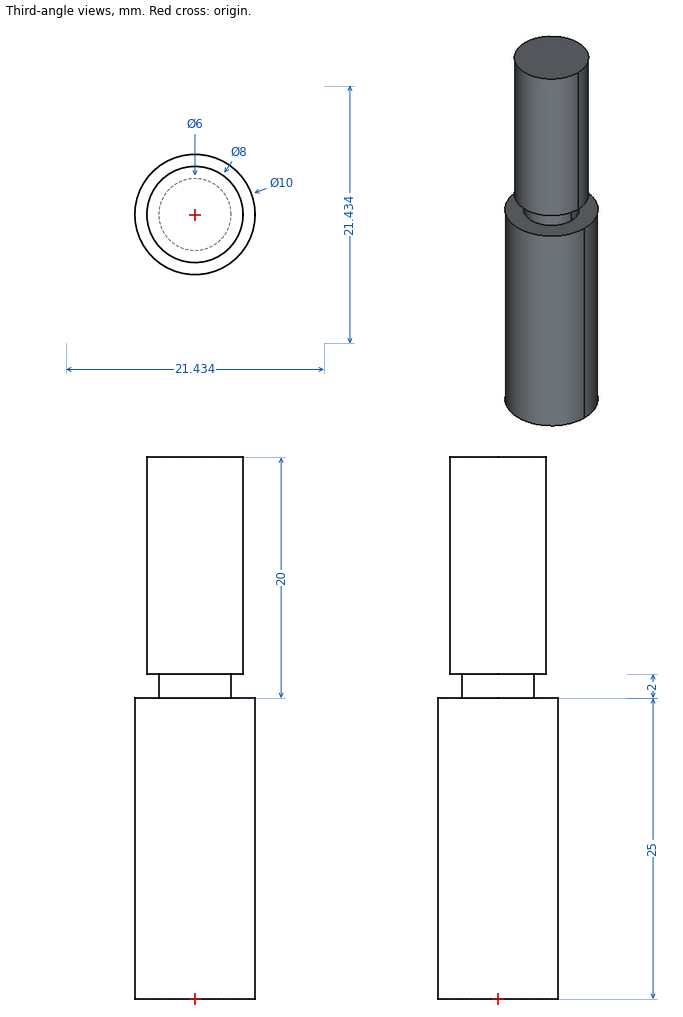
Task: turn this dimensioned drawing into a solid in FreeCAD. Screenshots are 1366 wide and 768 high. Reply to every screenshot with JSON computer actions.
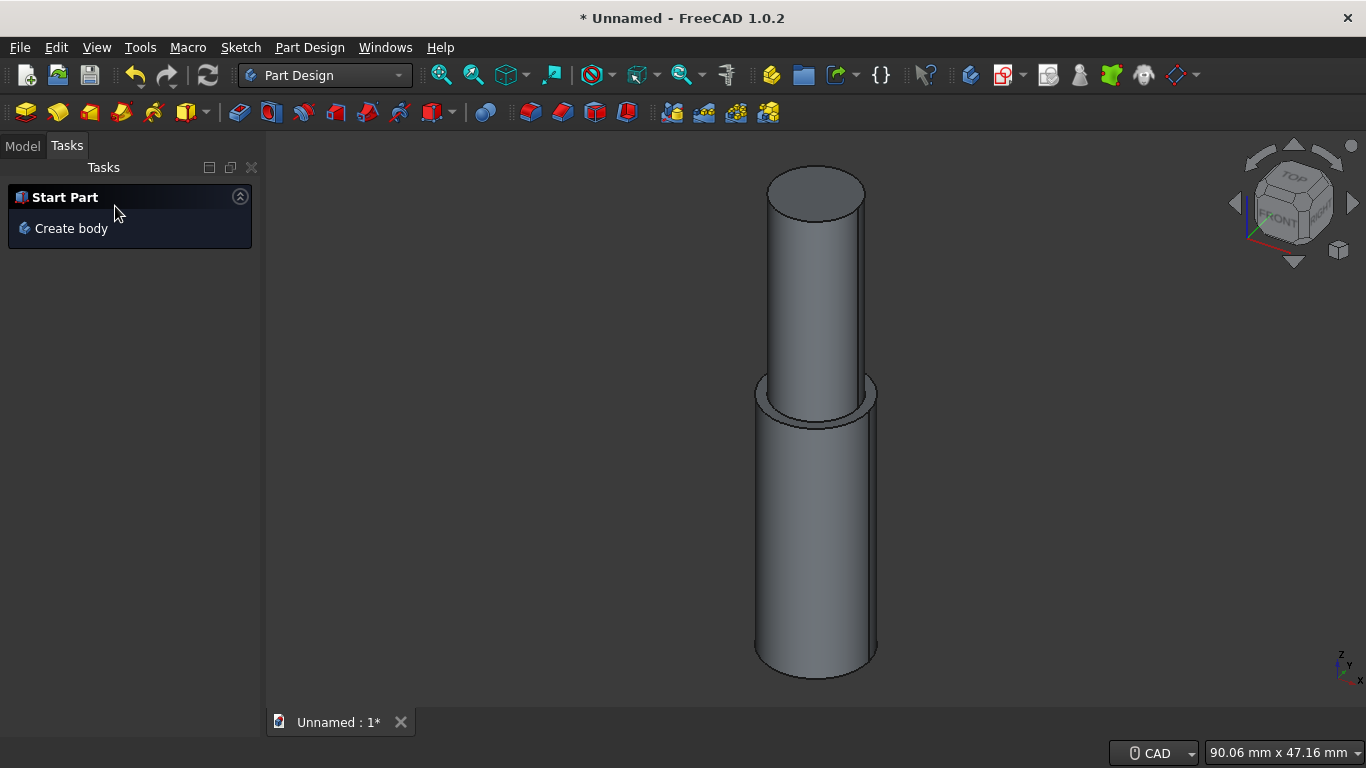
{"action": "scroll", "coordinate": [775, 414], "scroll_direction": "up", "scroll_amount": 4}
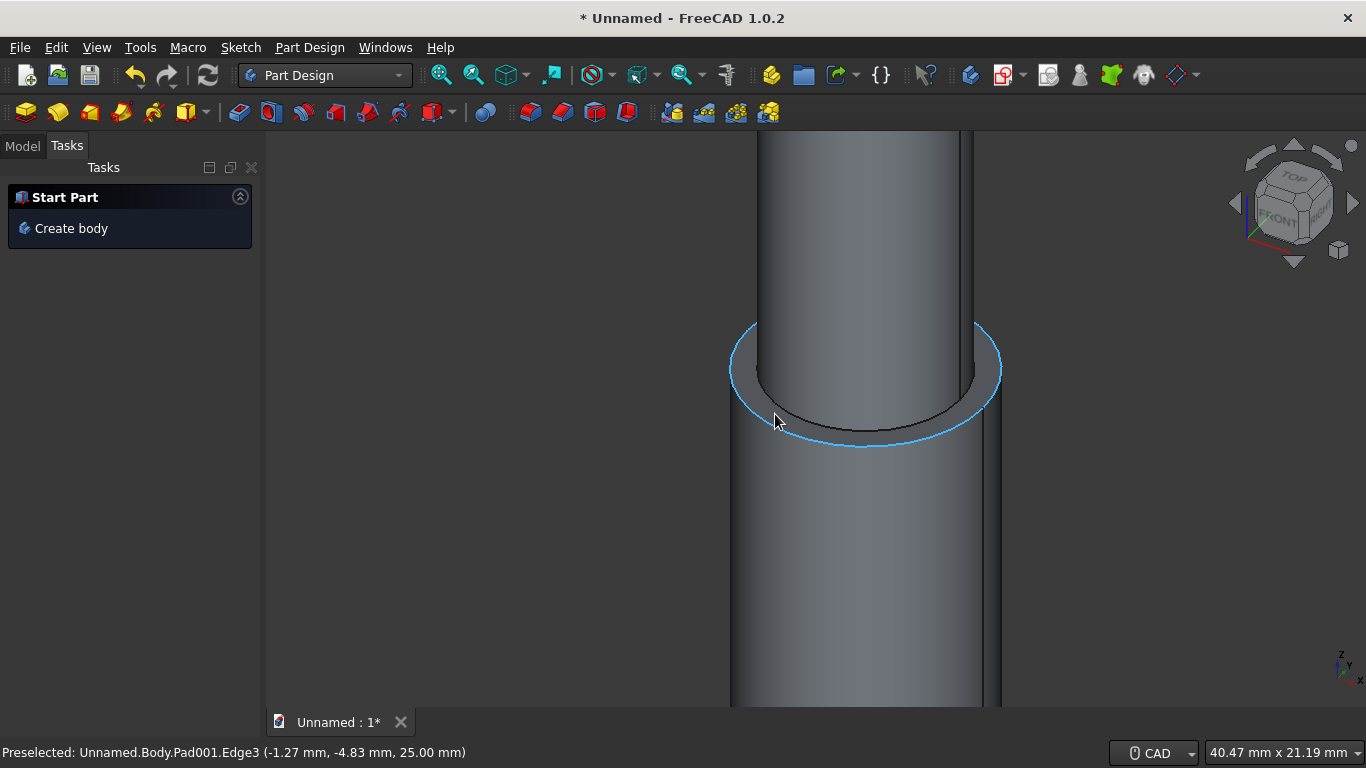
{"action": "left_click", "coordinate": [745, 354]}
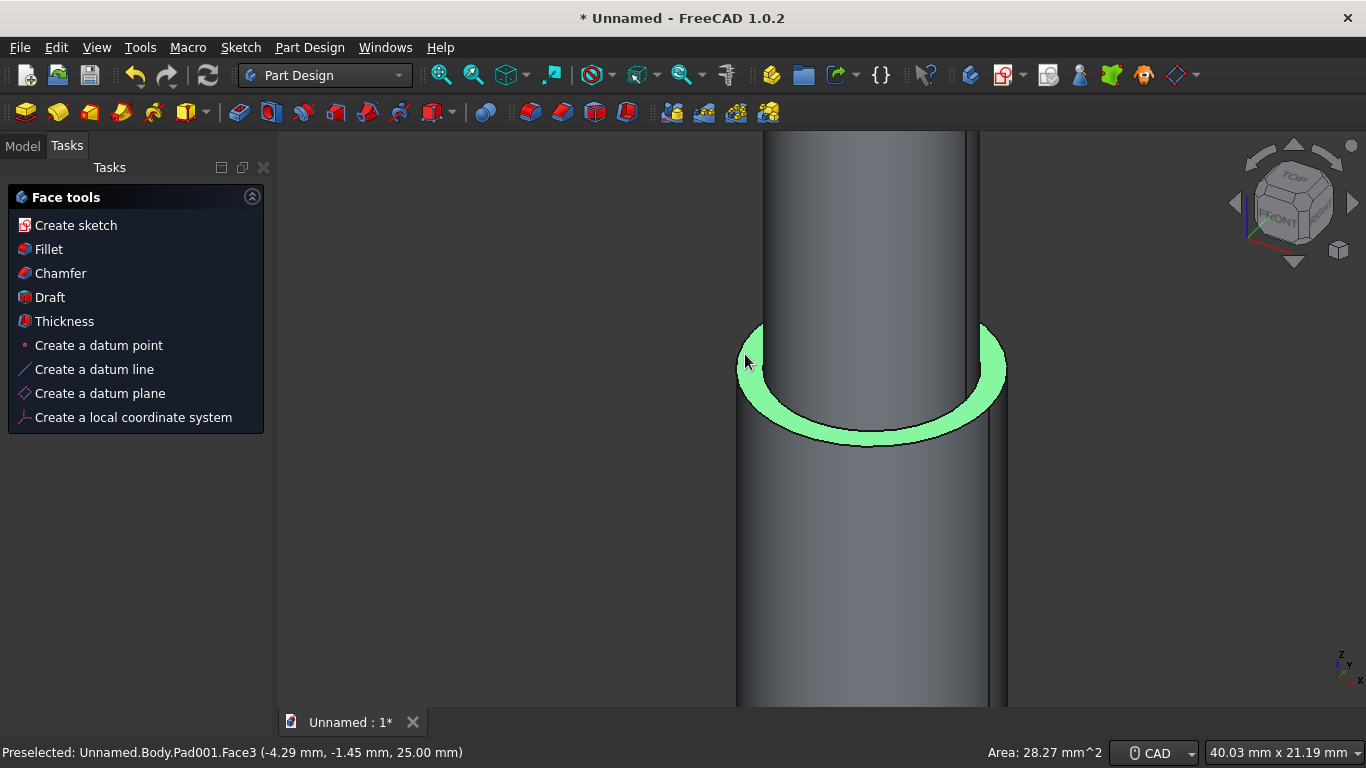
{"action": "left_click", "coordinate": [1004, 76]}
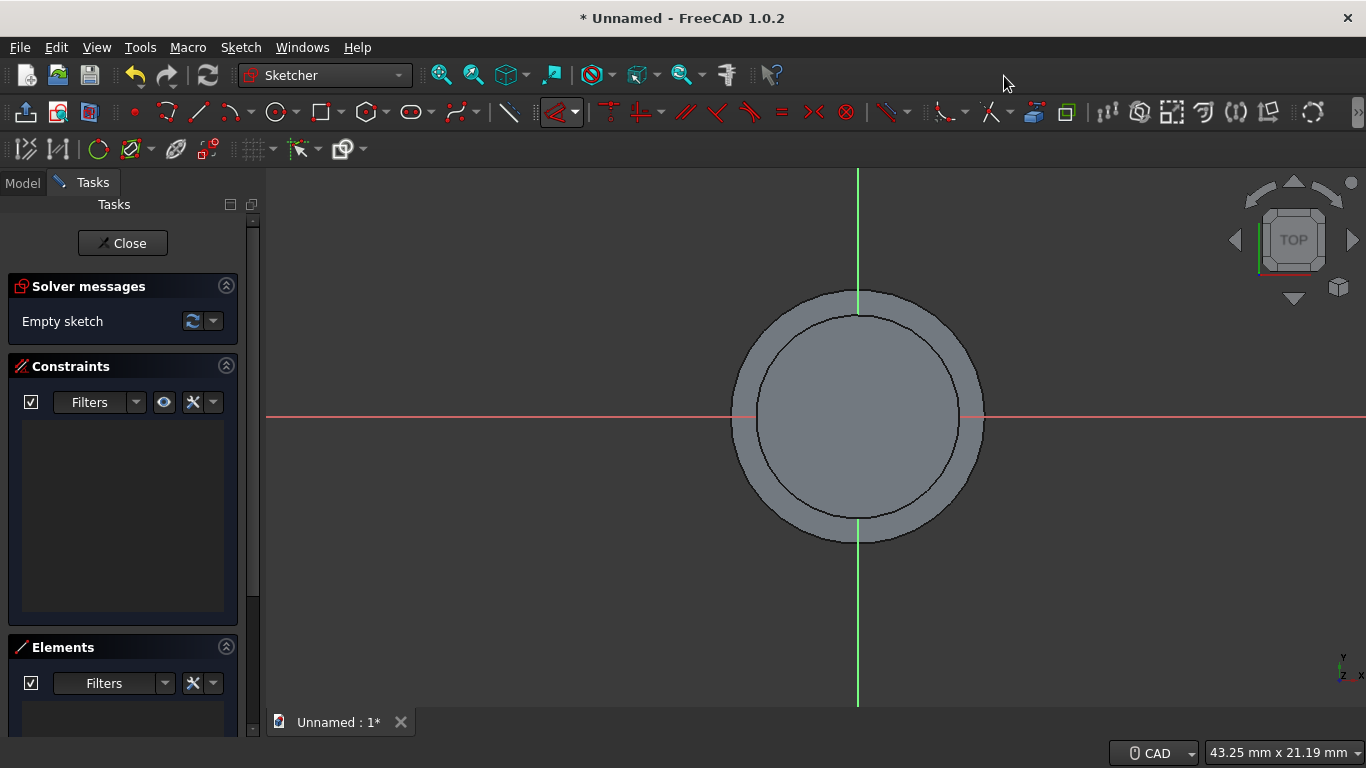
{"action": "scroll", "coordinate": [523, 480], "scroll_direction": "down", "scroll_amount": 2}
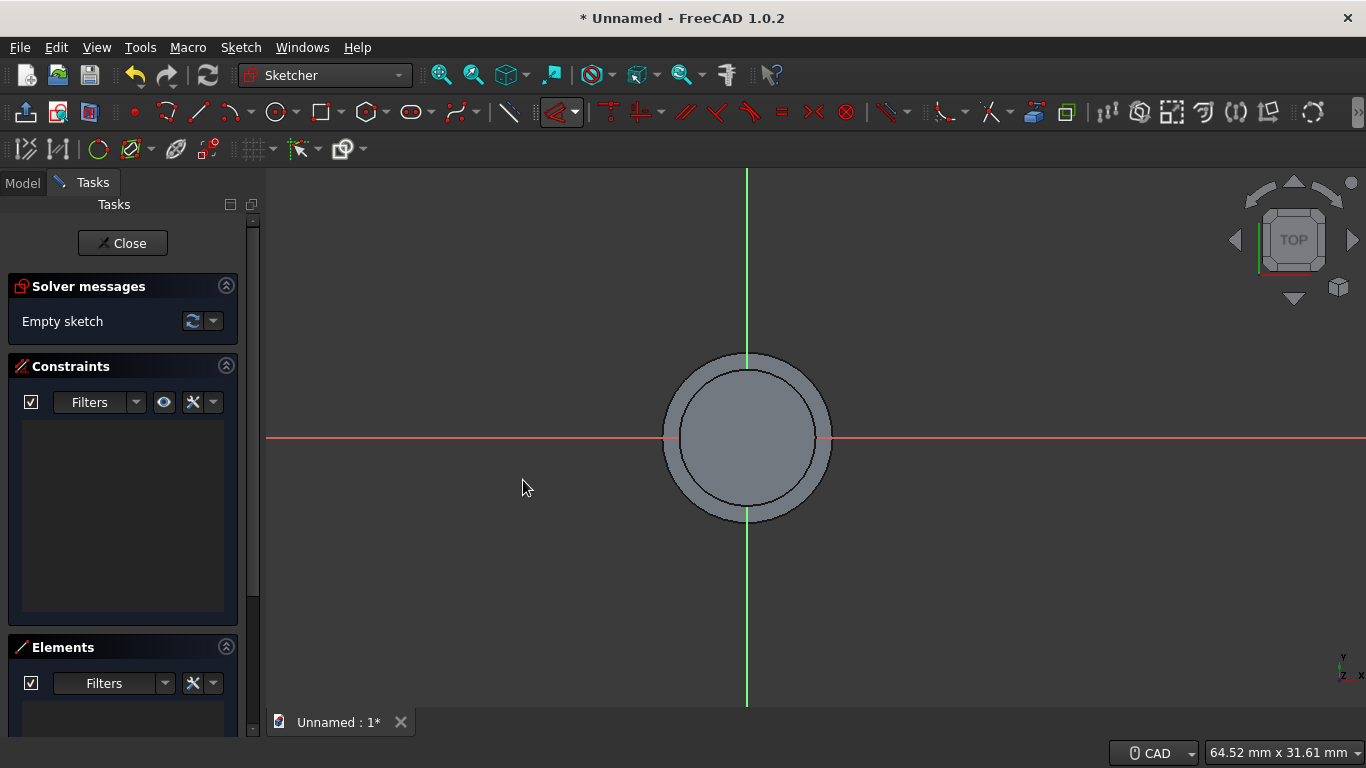
{"action": "key", "text": "g v"}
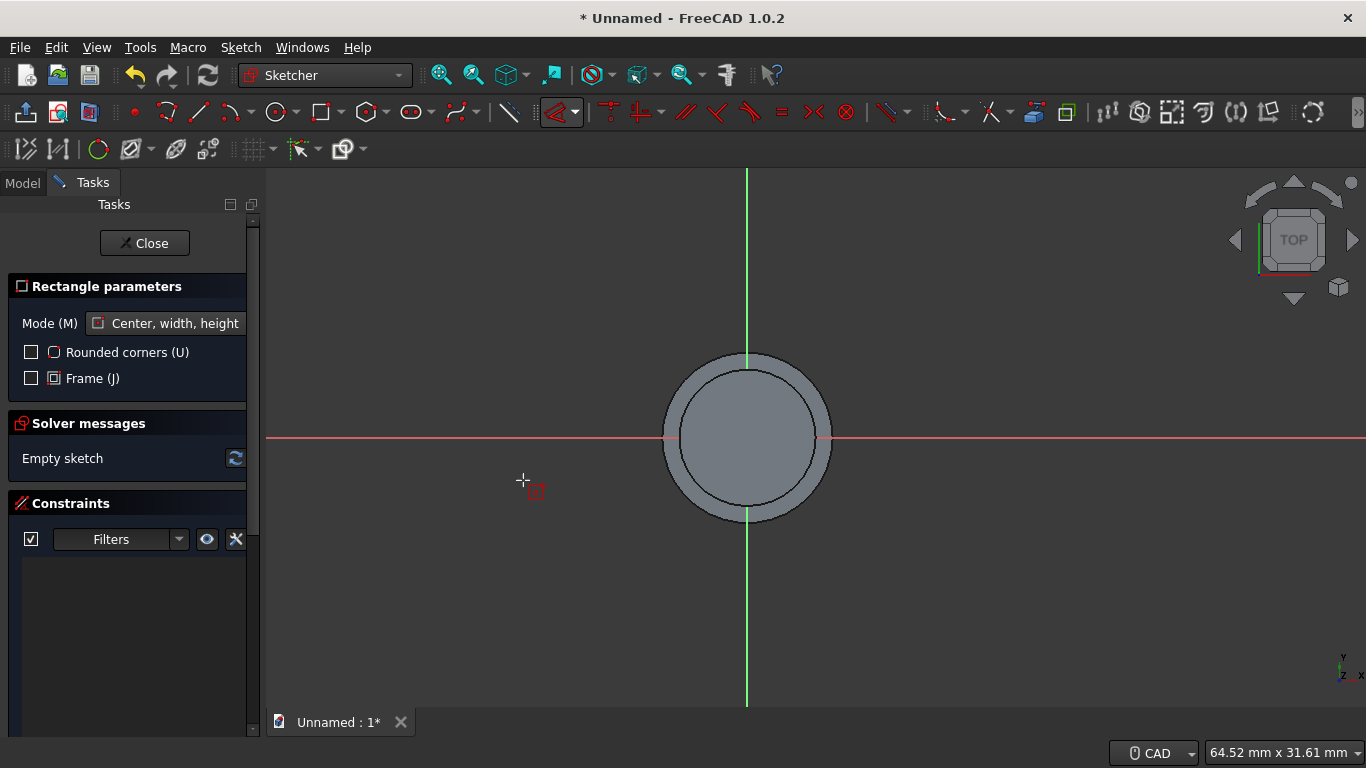
{"action": "left_click", "coordinate": [747, 438]}
{"action": "left_click", "coordinate": [930, 255]}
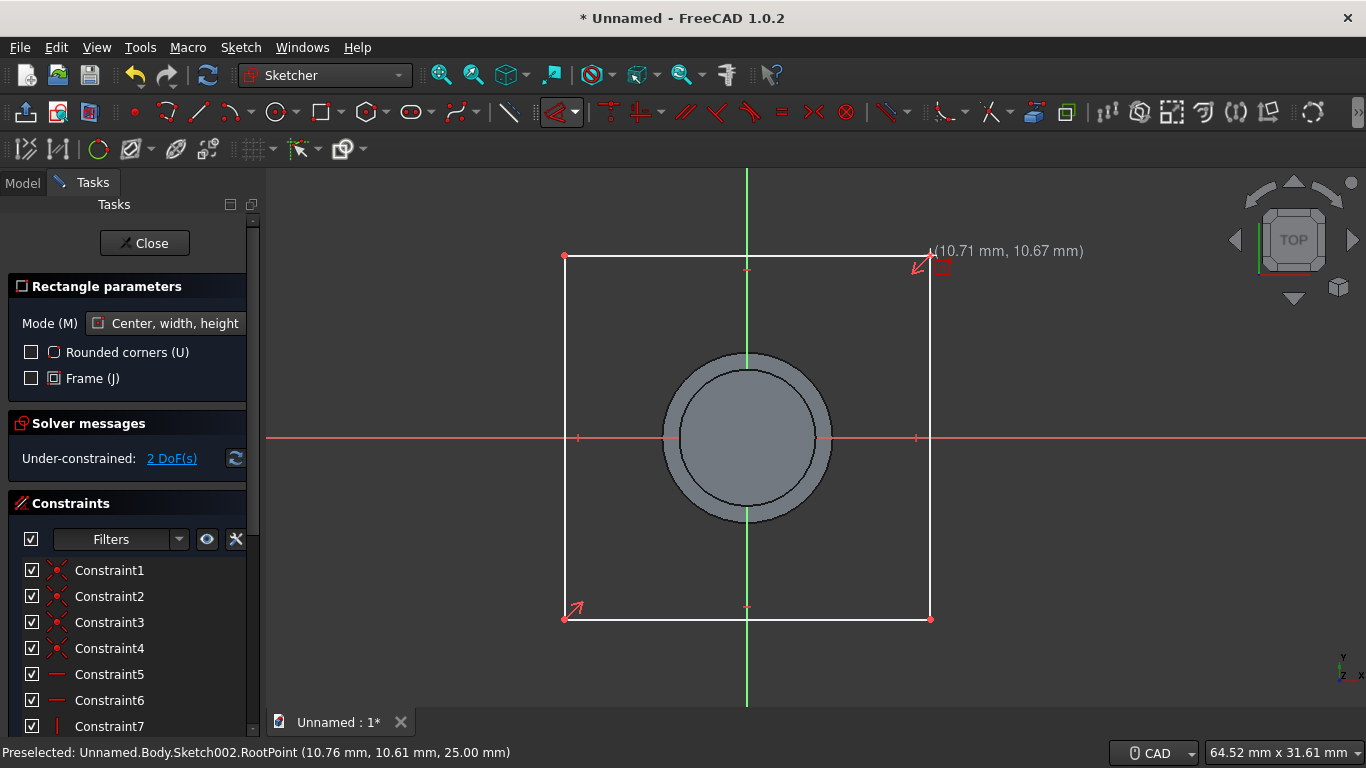
{"action": "left_click", "coordinate": [276, 112]}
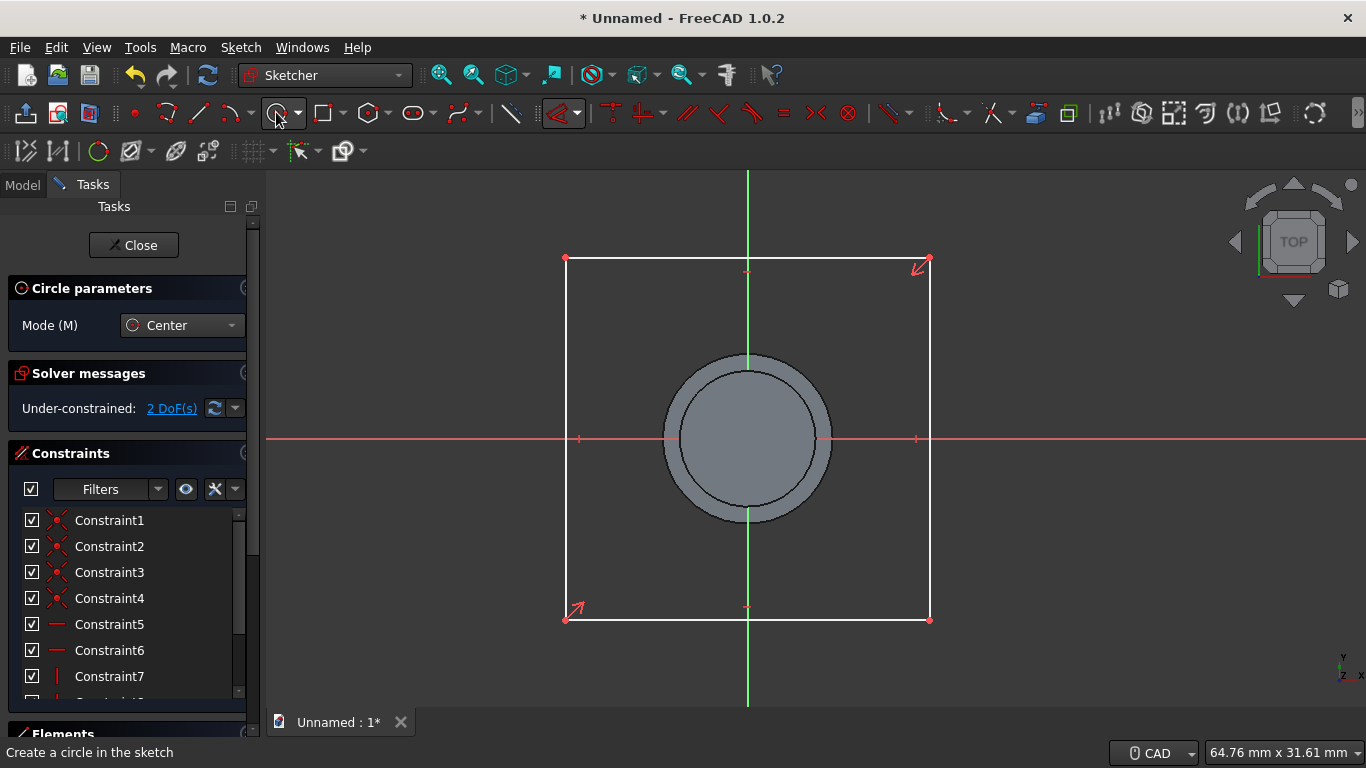
{"action": "left_click", "coordinate": [748, 439]}
{"action": "left_click", "coordinate": [784, 403]}
{"action": "key", "text": "Escape"}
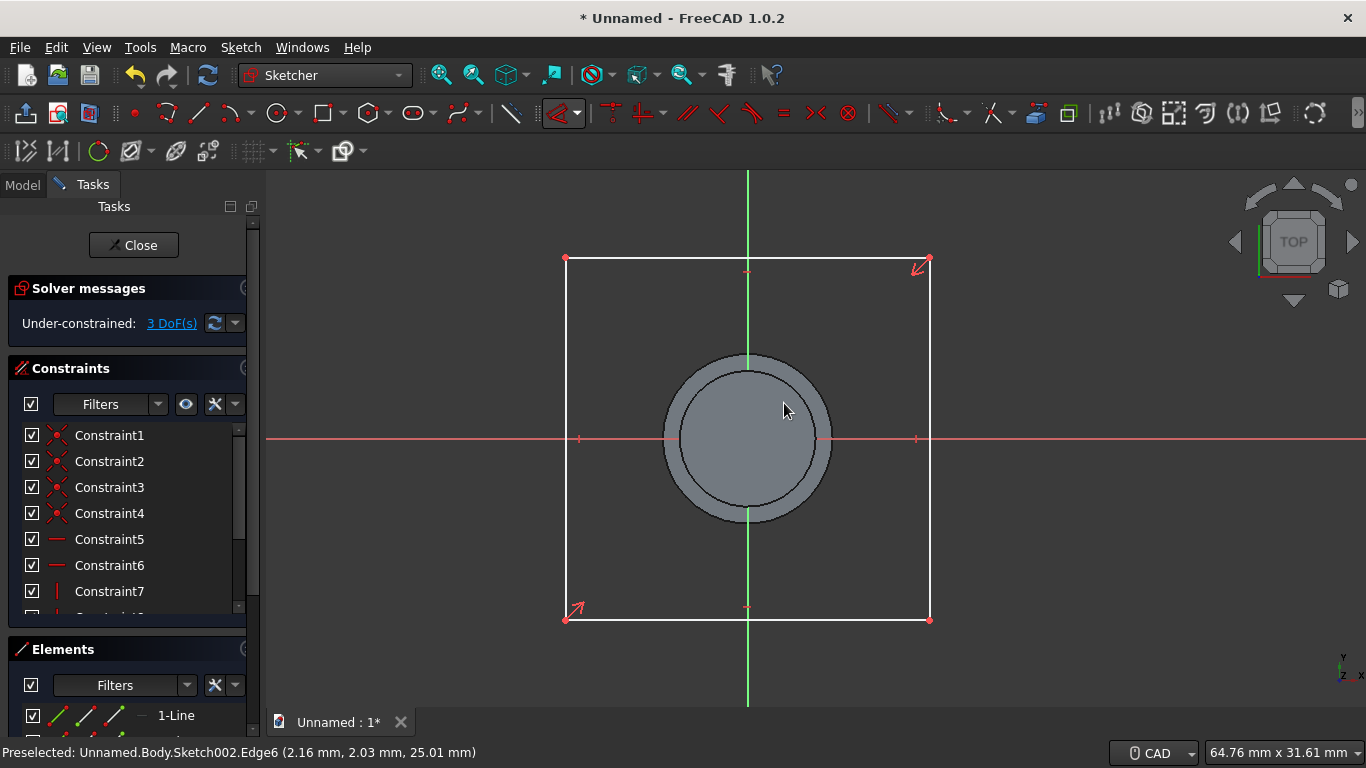
{"action": "left_click", "coordinate": [783, 403]}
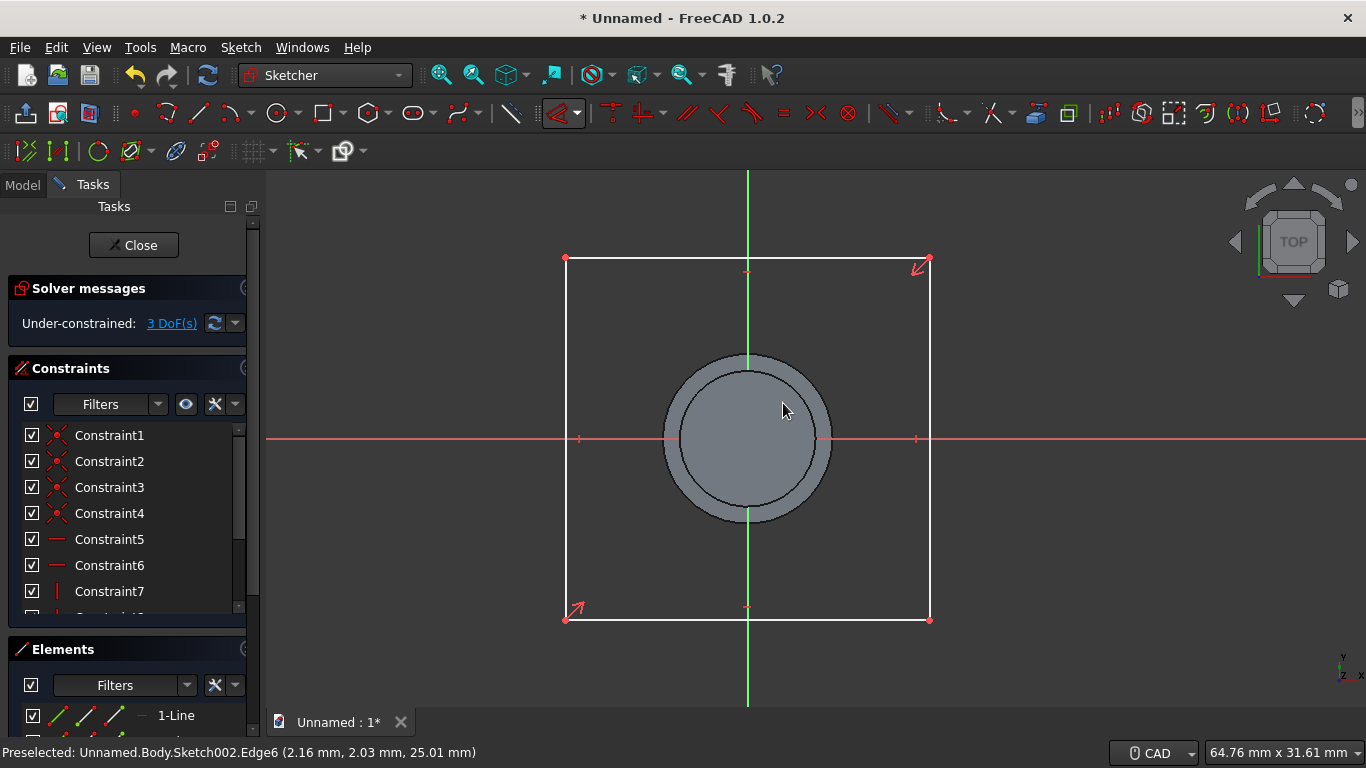
{"action": "key", "text": "k o"}